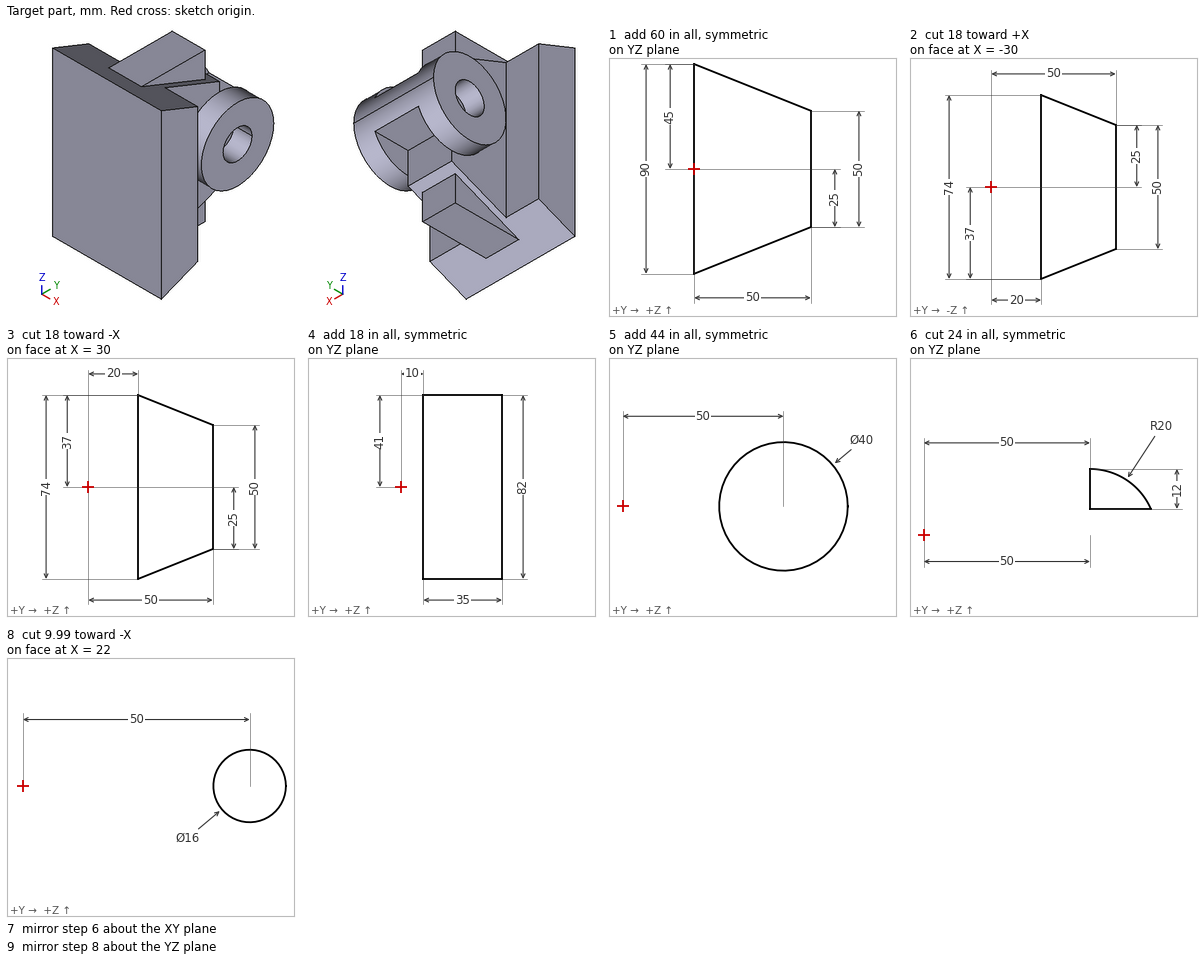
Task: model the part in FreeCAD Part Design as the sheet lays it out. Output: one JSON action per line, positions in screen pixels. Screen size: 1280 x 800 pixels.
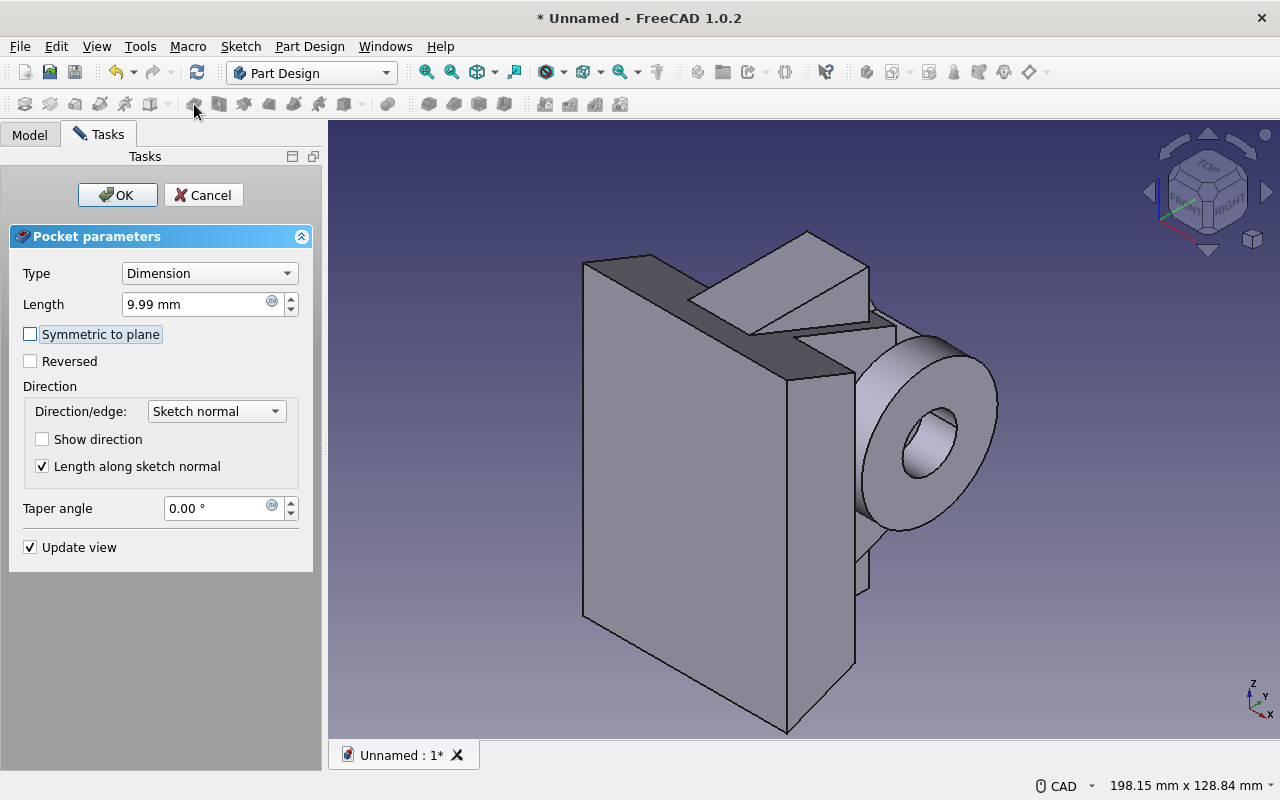
{"action": "left_click", "coordinate": [118, 195]}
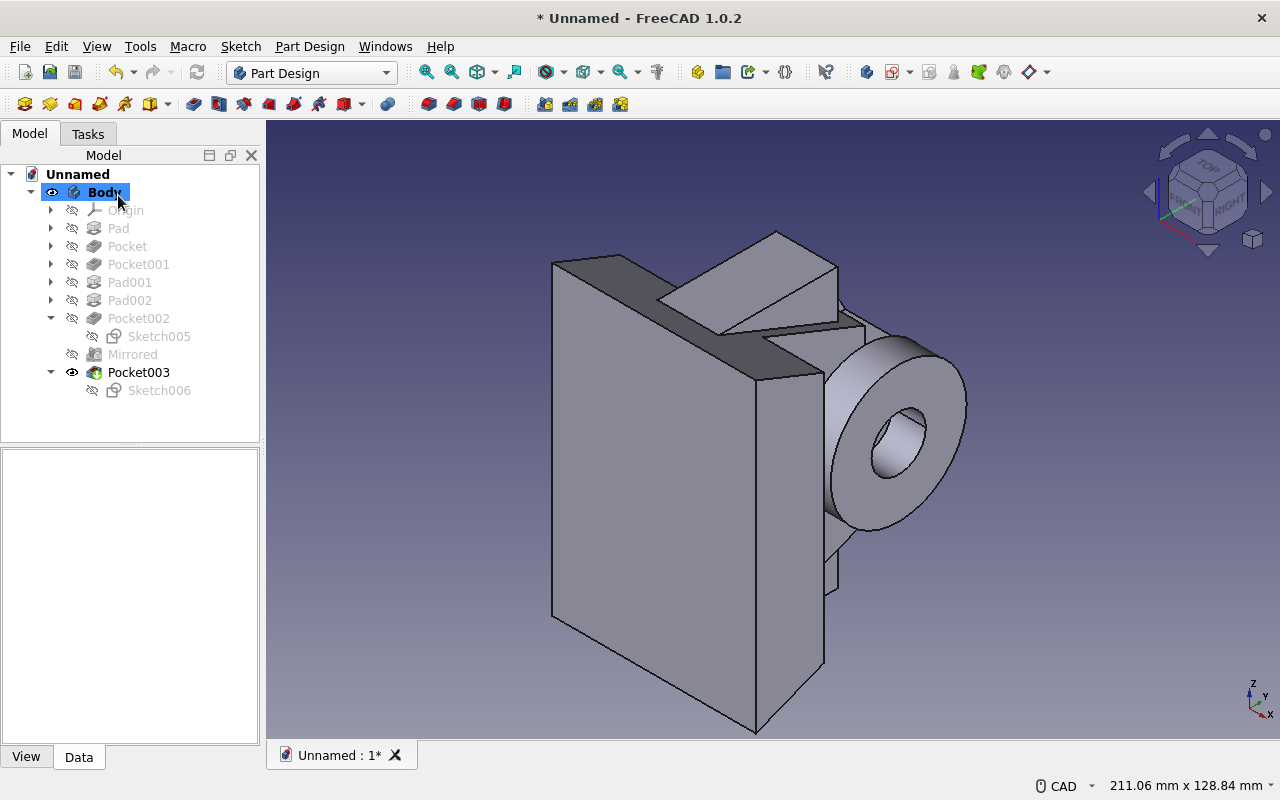
{"action": "left_click", "coordinate": [117, 372]}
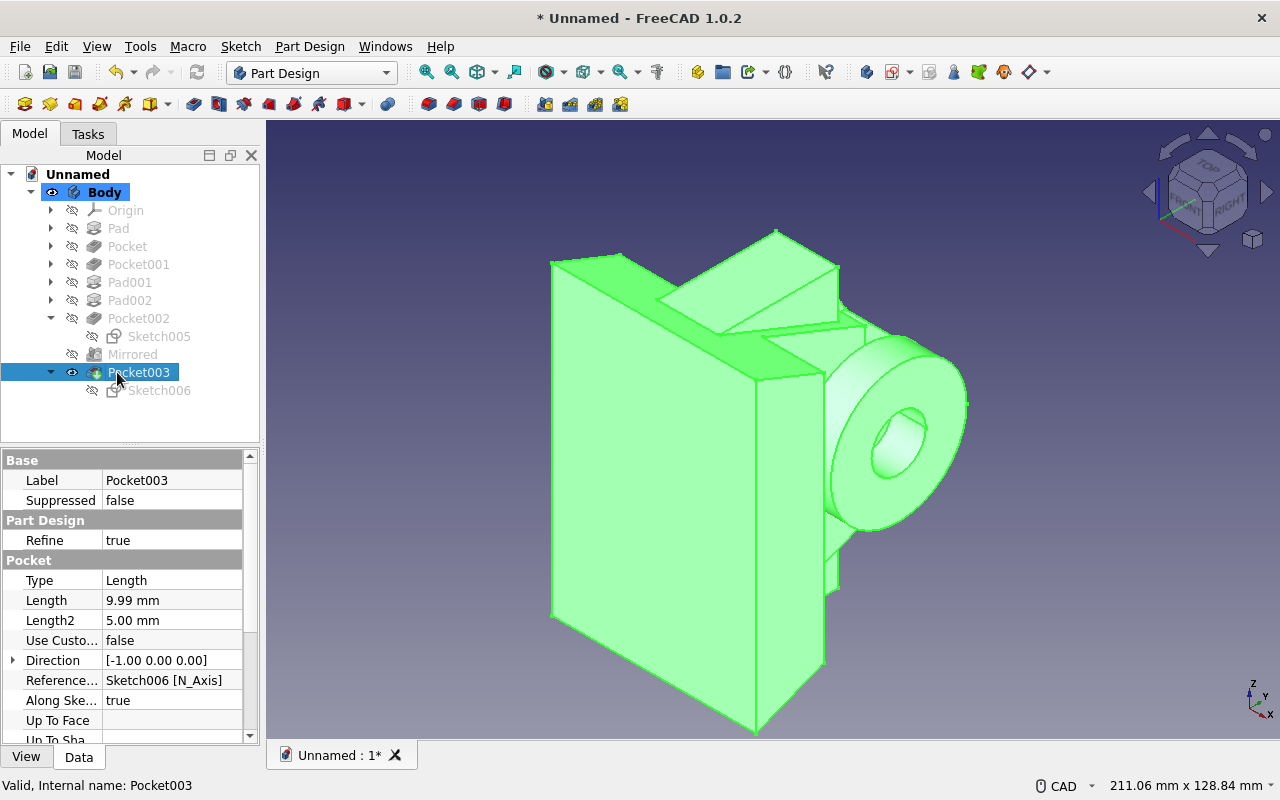
{"action": "left_click", "coordinate": [545, 104]}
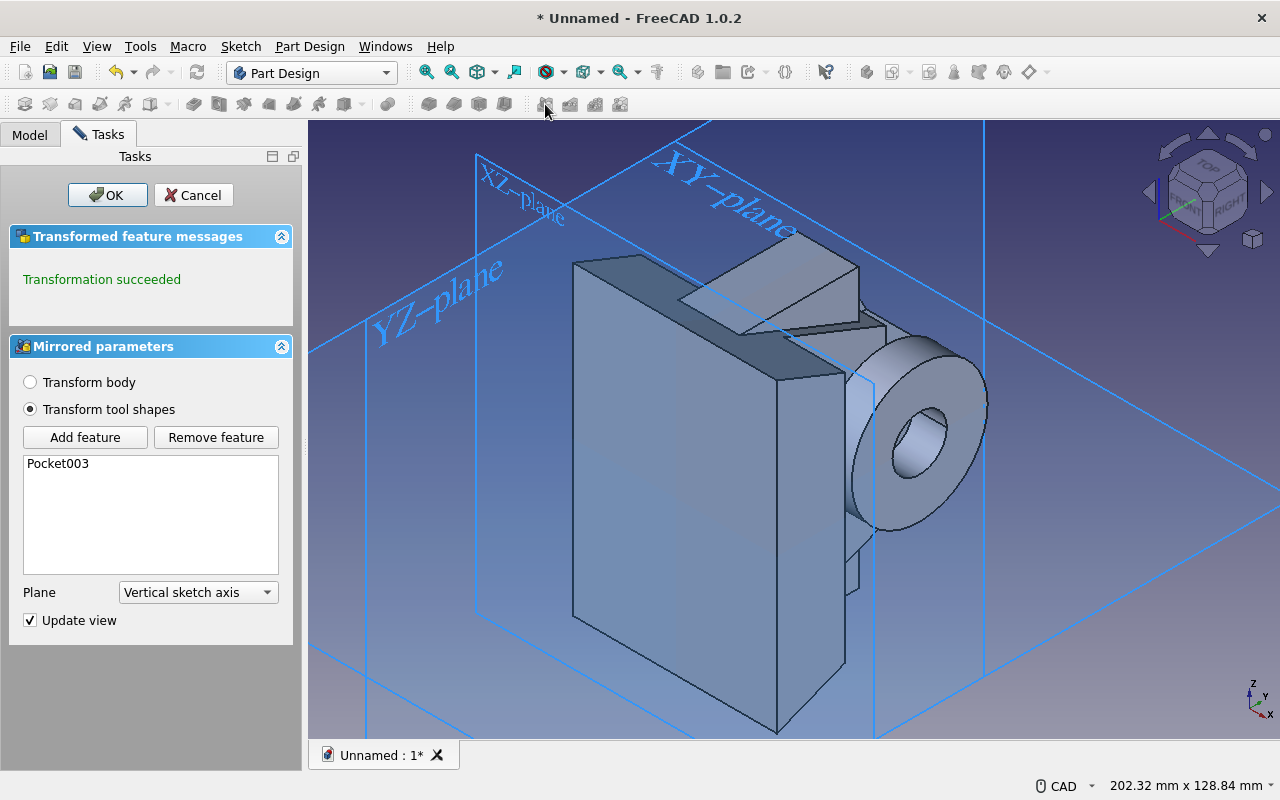
{"action": "left_click", "coordinate": [199, 592]}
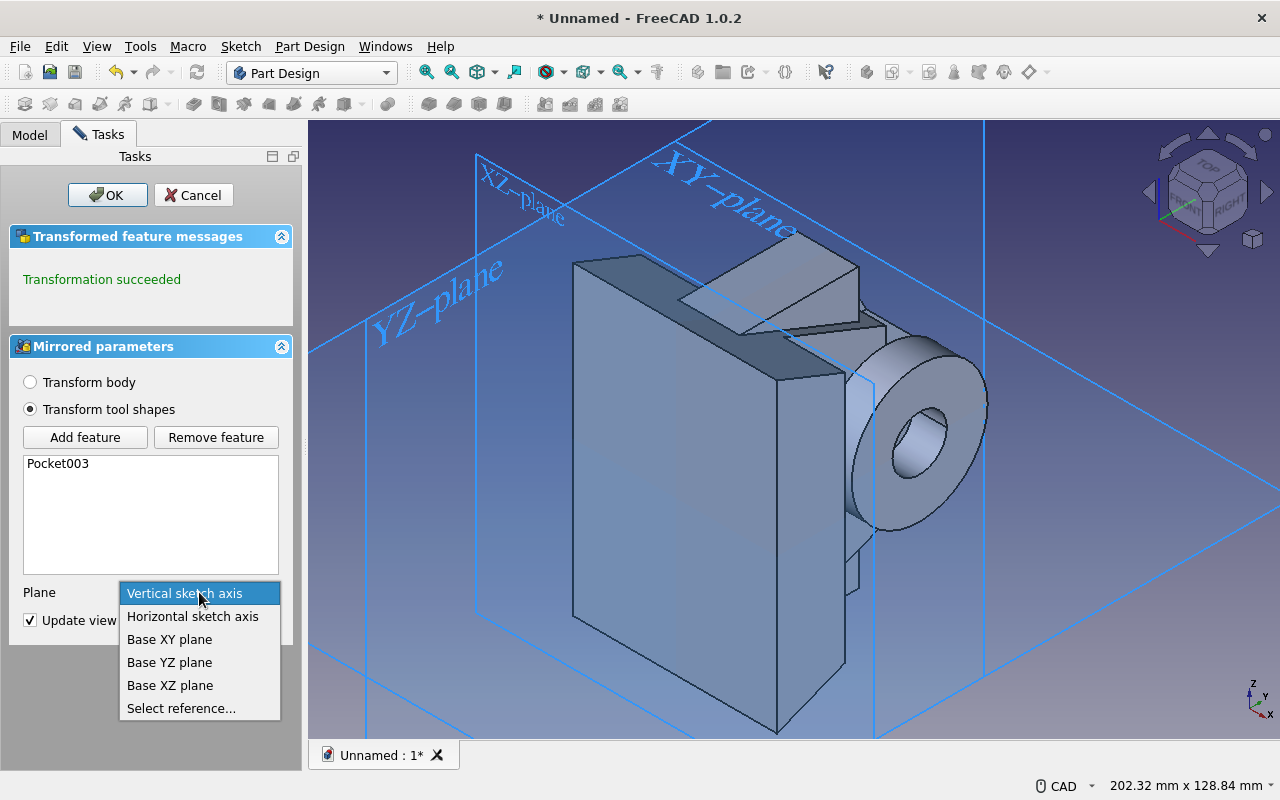
{"action": "left_click", "coordinate": [198, 662]}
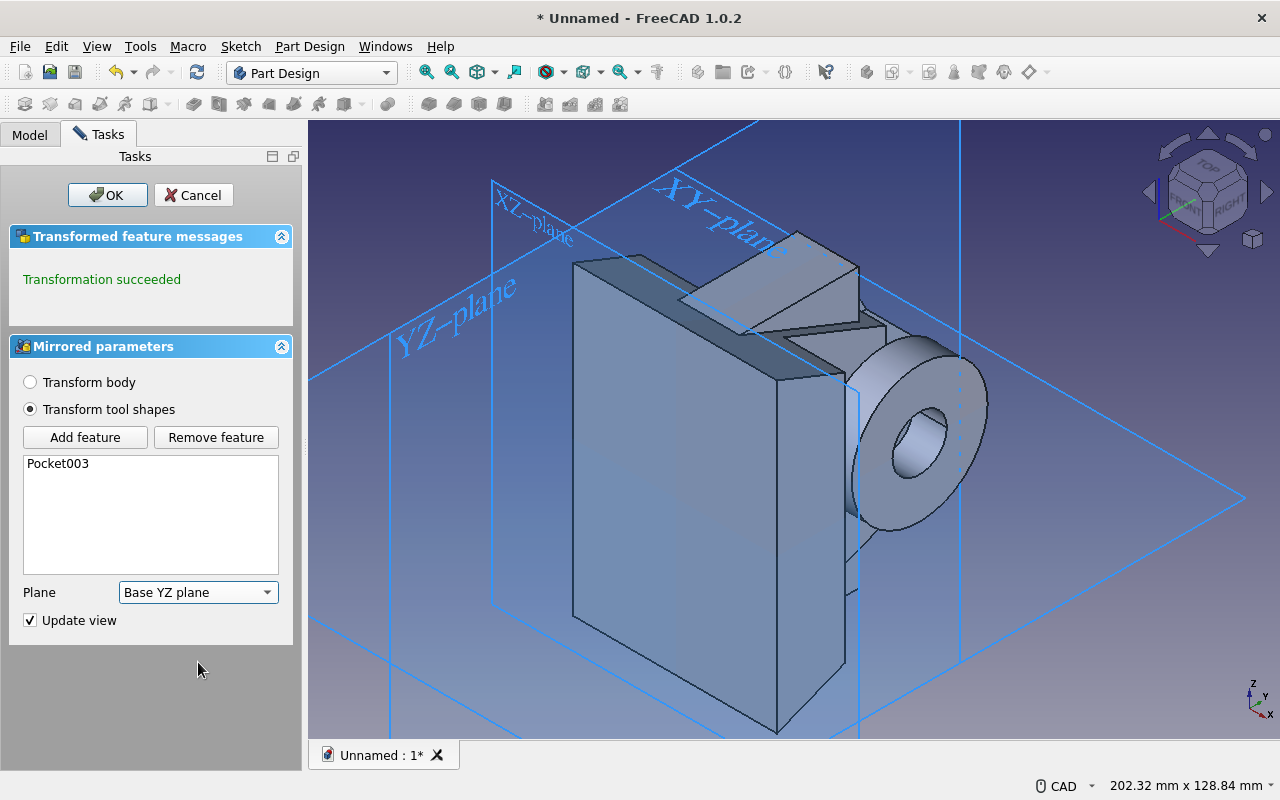
{"action": "left_click", "coordinate": [108, 195]}